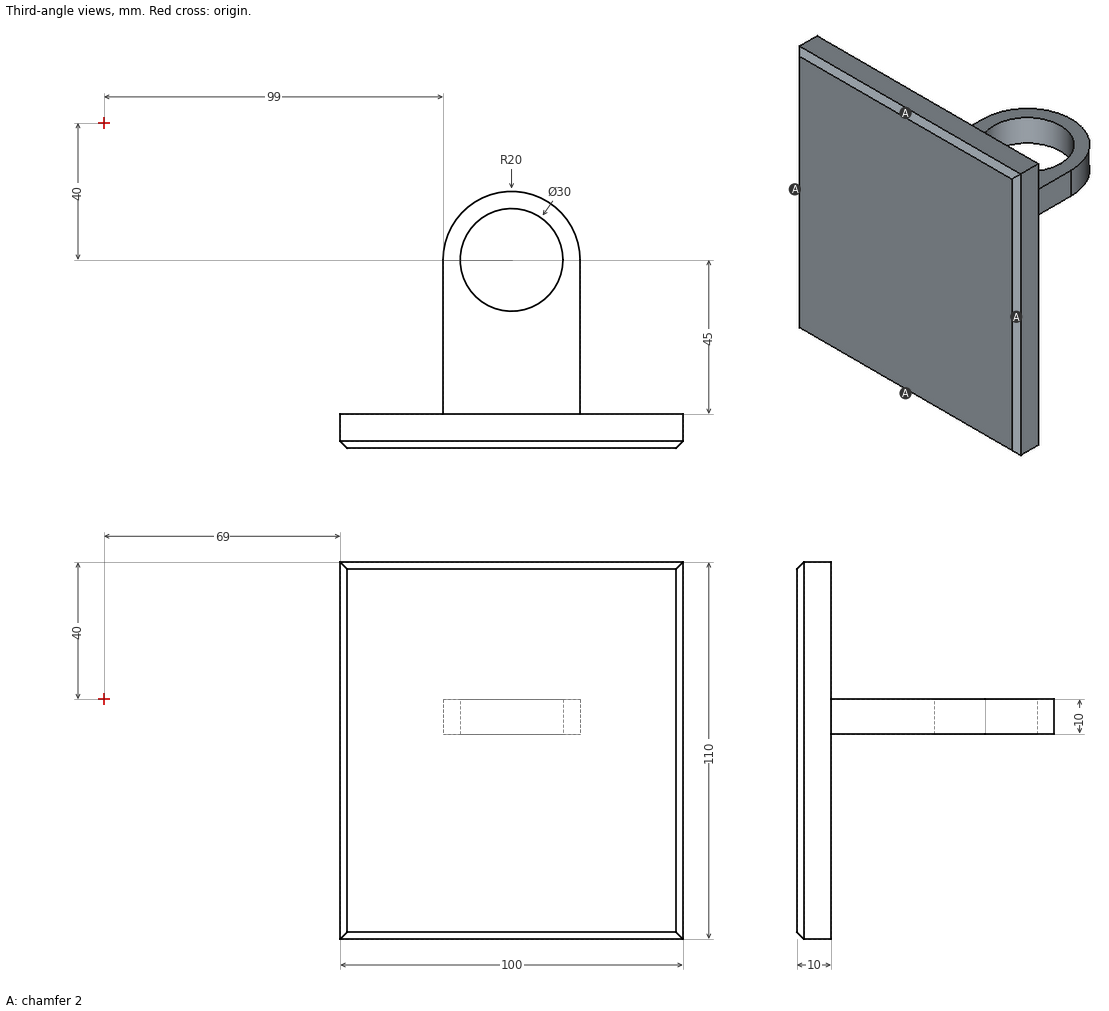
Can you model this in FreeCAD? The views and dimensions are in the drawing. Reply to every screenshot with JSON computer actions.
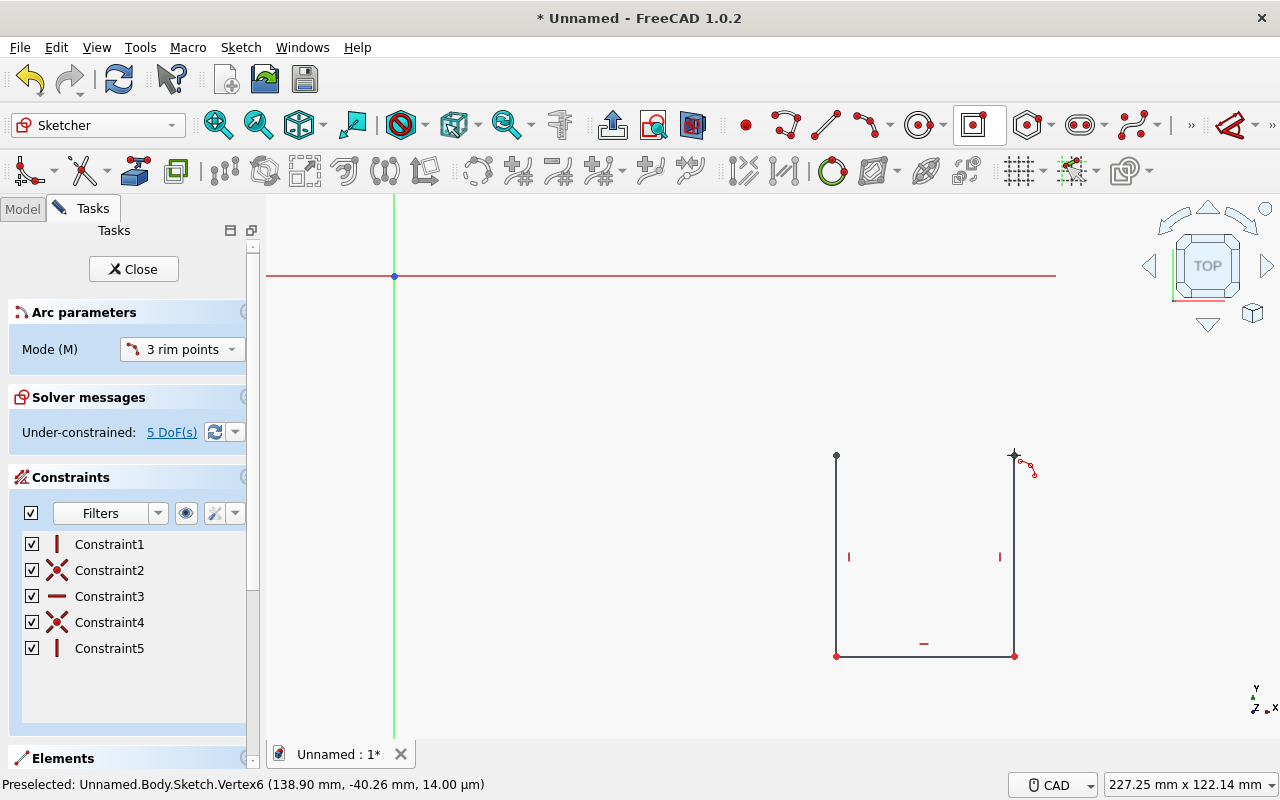
{"action": "left_click", "coordinate": [1014, 456]}
{"action": "left_click", "coordinate": [836, 456]}
{"action": "left_click", "coordinate": [925, 366]}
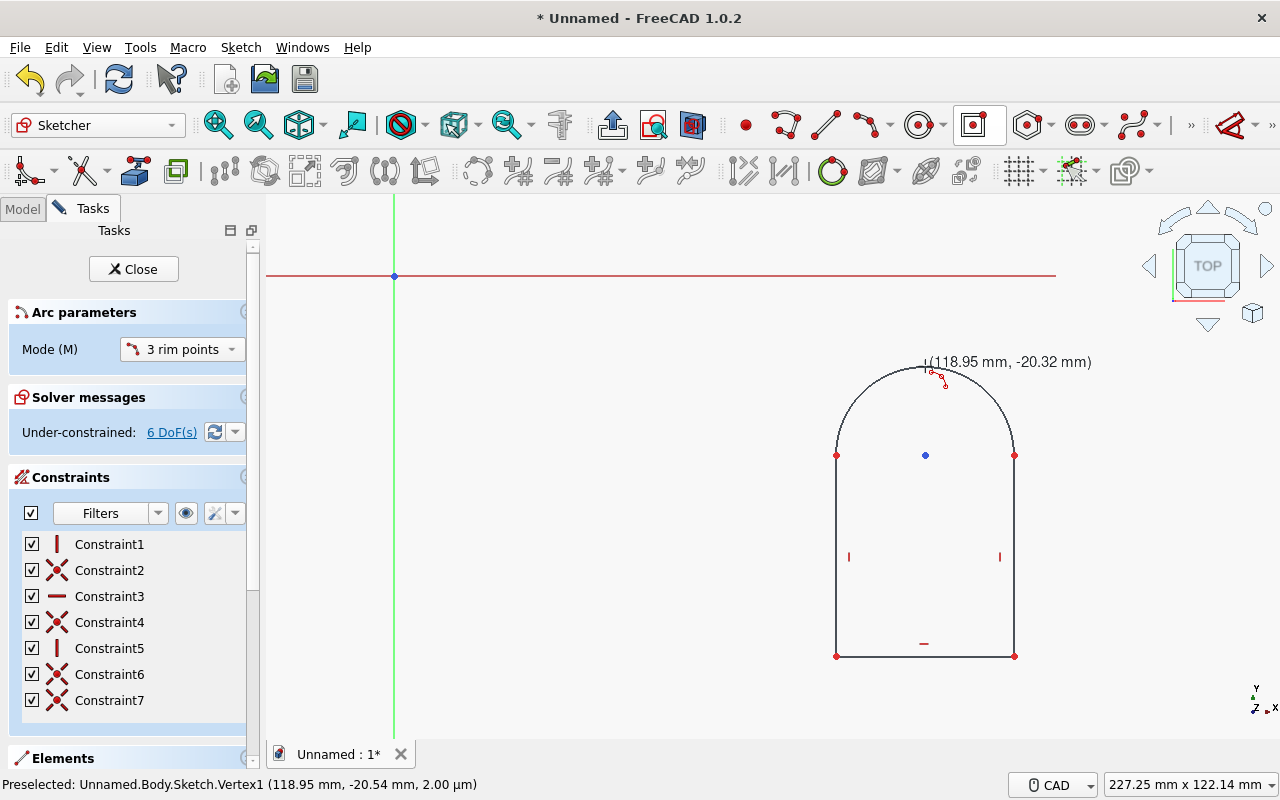
{"action": "left_click", "coordinate": [920, 126]}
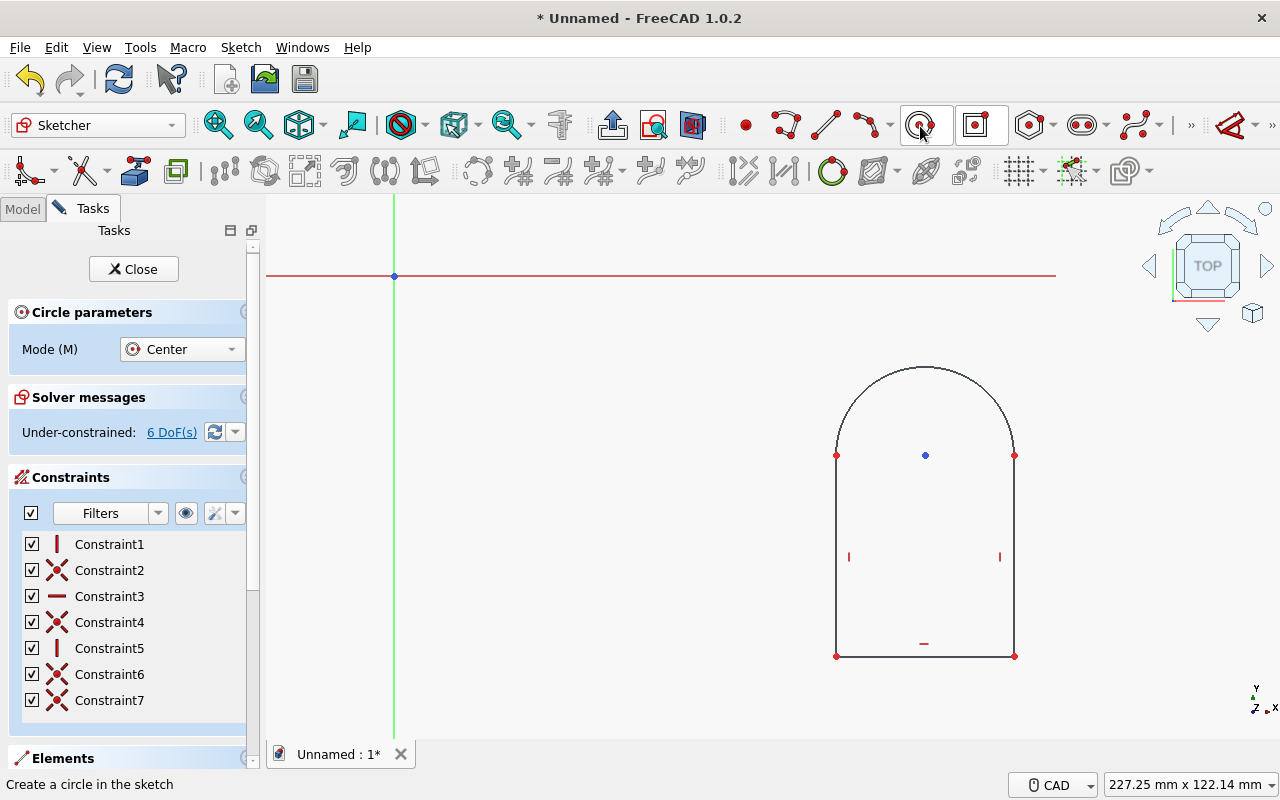
{"action": "left_click", "coordinate": [925, 455]}
{"action": "mouse_move", "coordinate": [973, 407]}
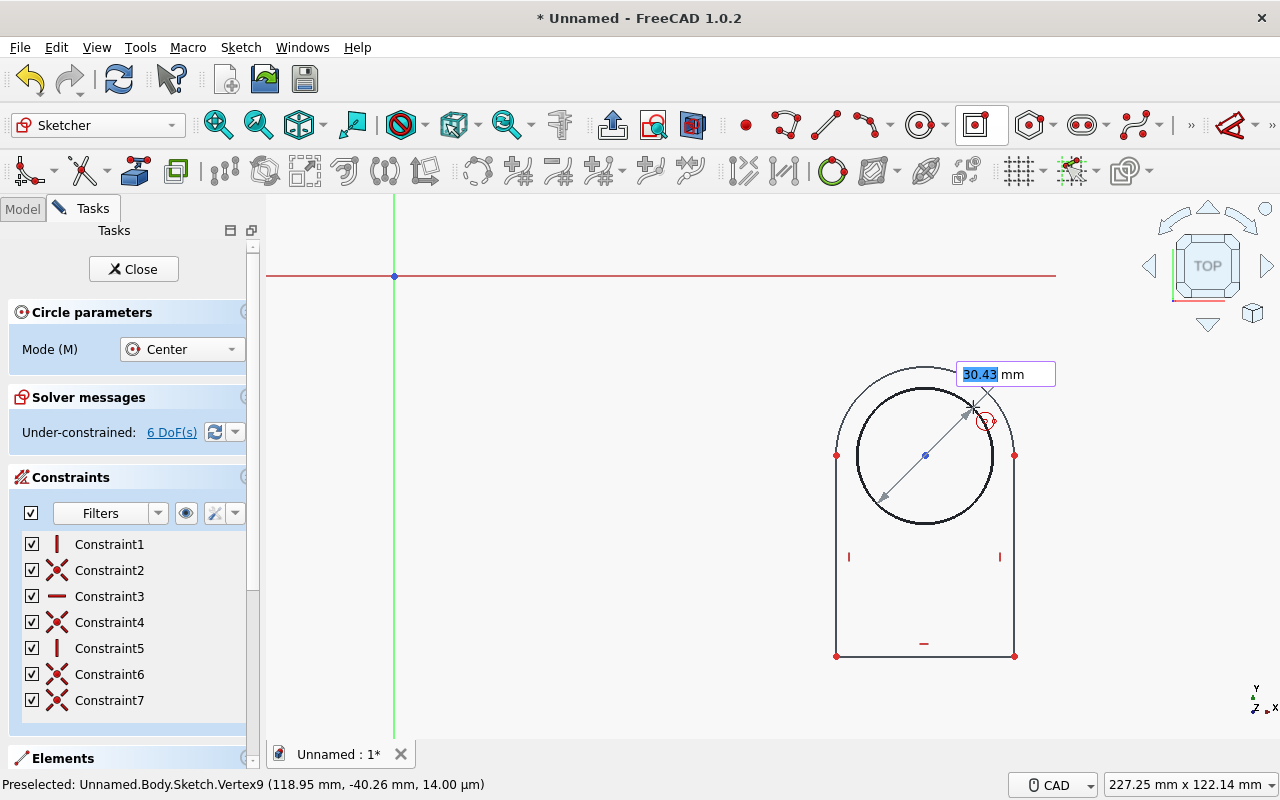
{"action": "type", "text": "30"}
{"action": "key", "text": "Return"}
{"action": "key", "text": "Escape"}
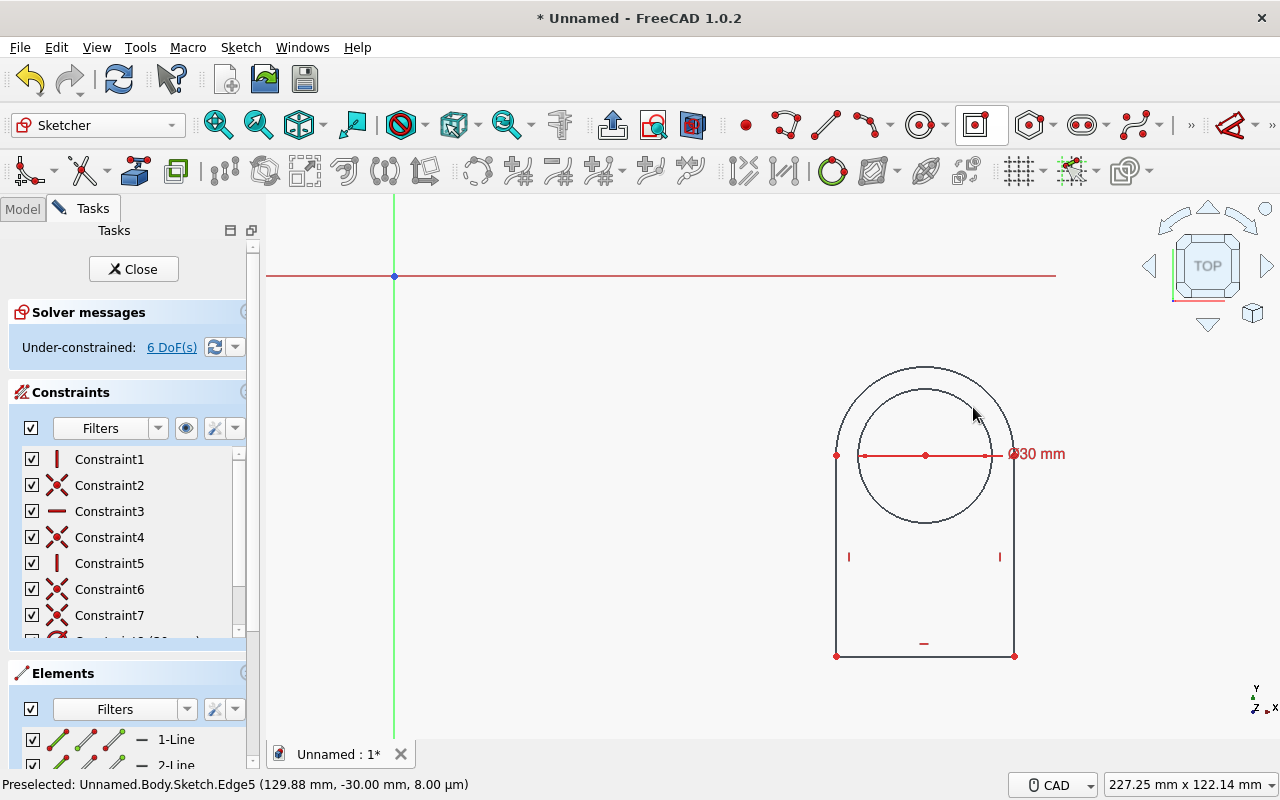
{"action": "left_click", "coordinate": [836, 516]}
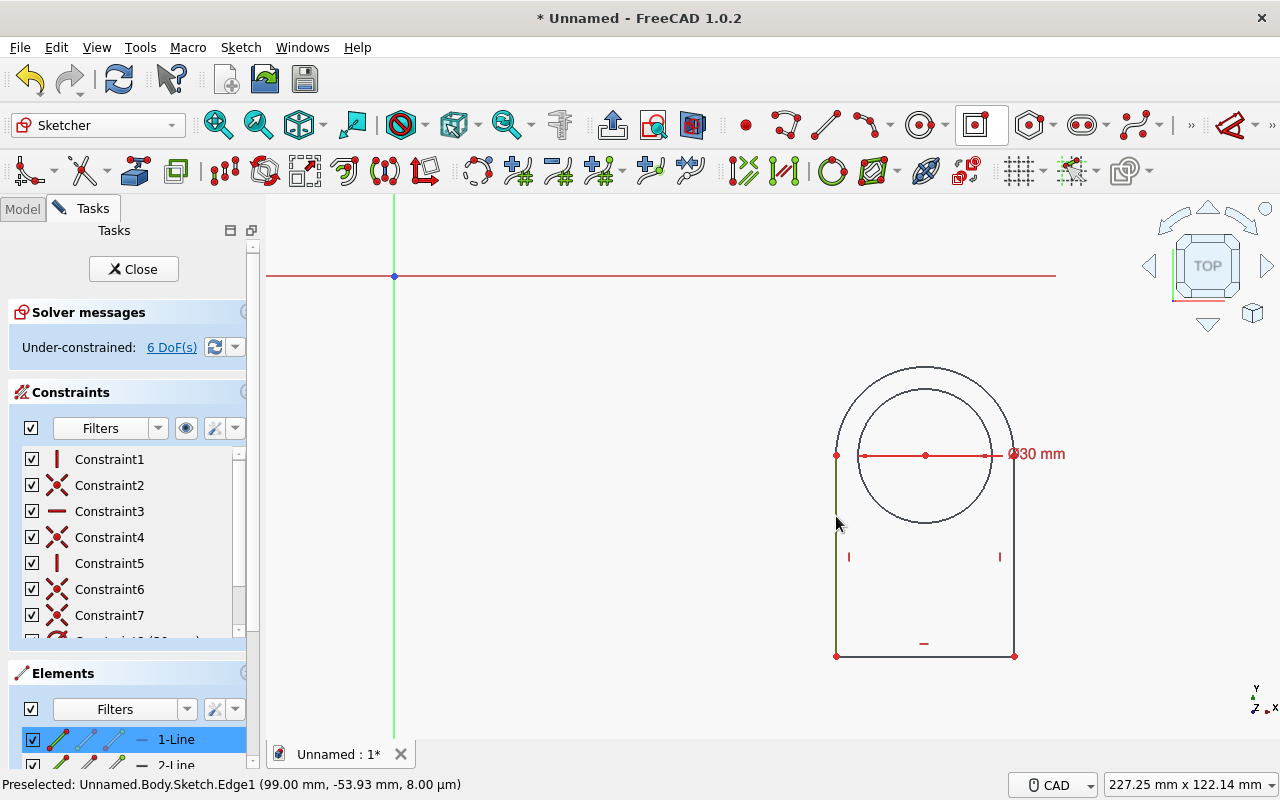
{"action": "left_click", "coordinate": [977, 384]}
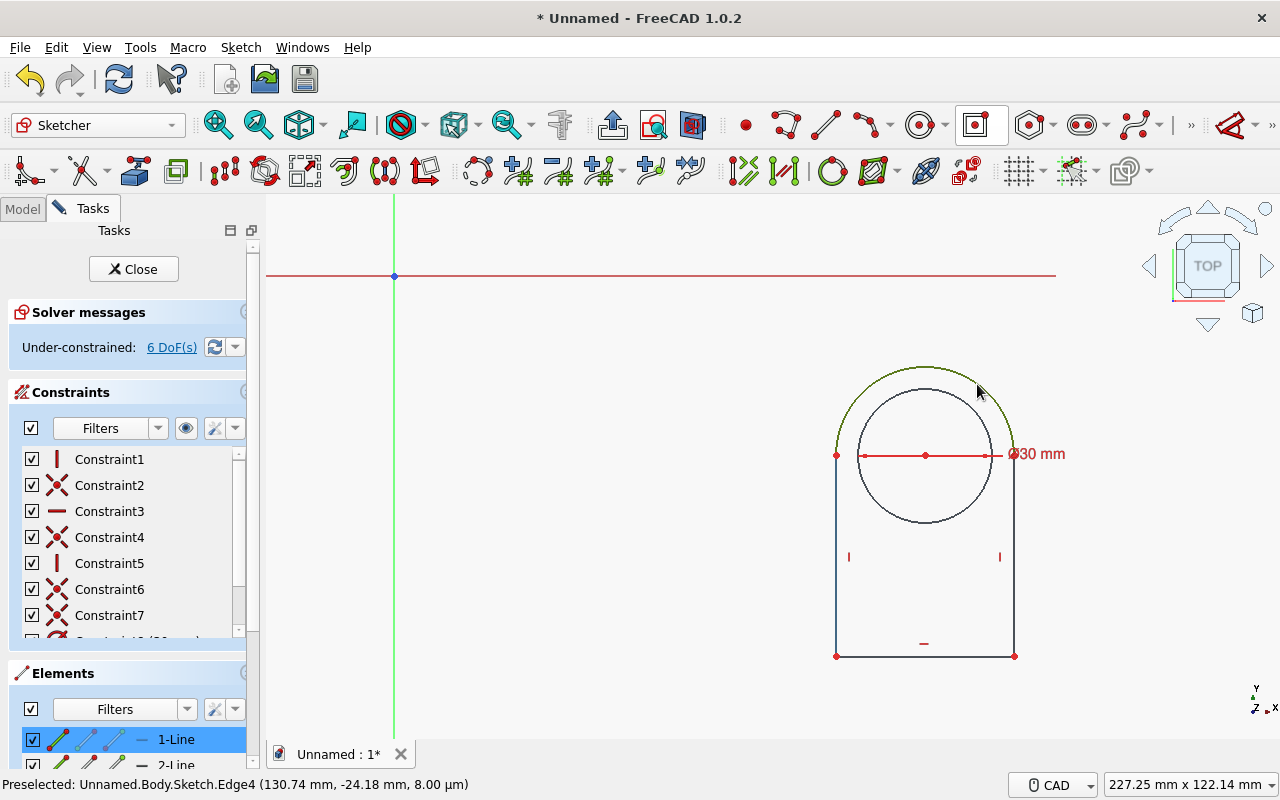
{"action": "key", "text": "t"}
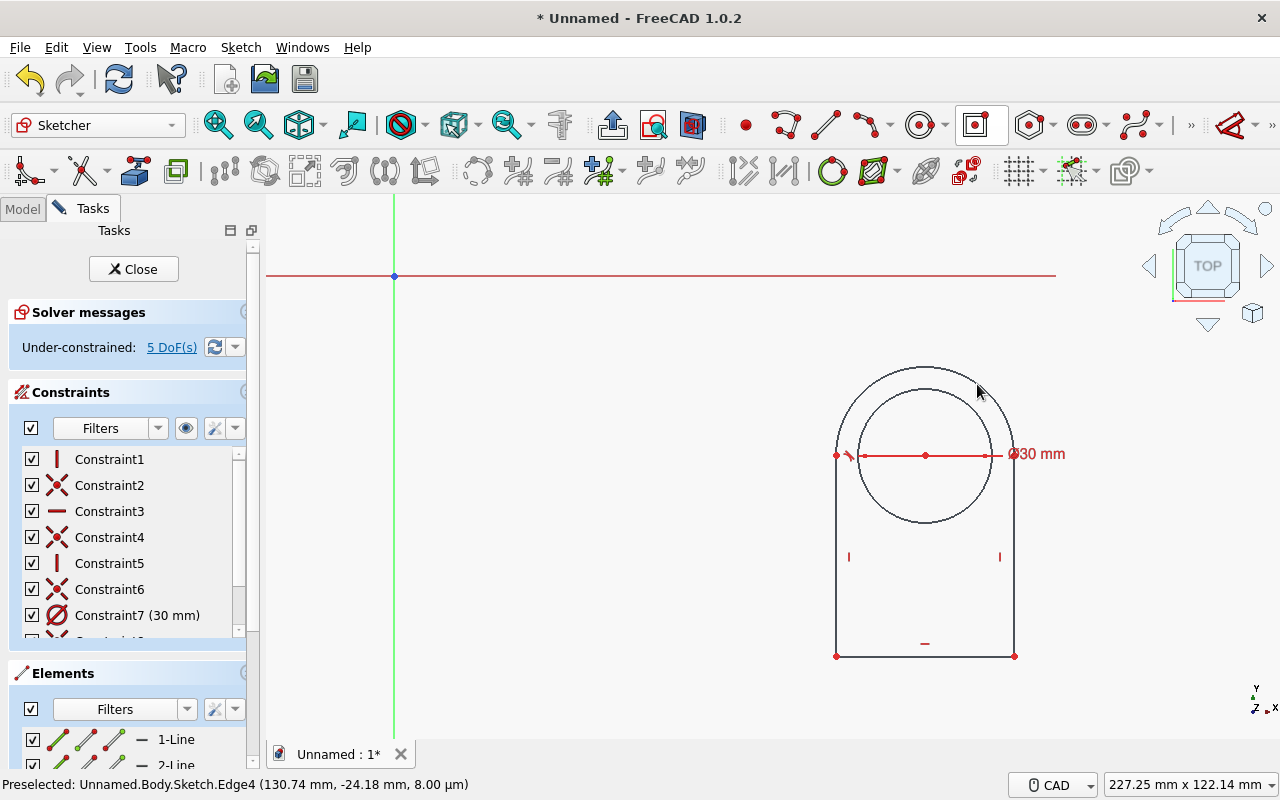
{"action": "left_click", "coordinate": [1014, 597]}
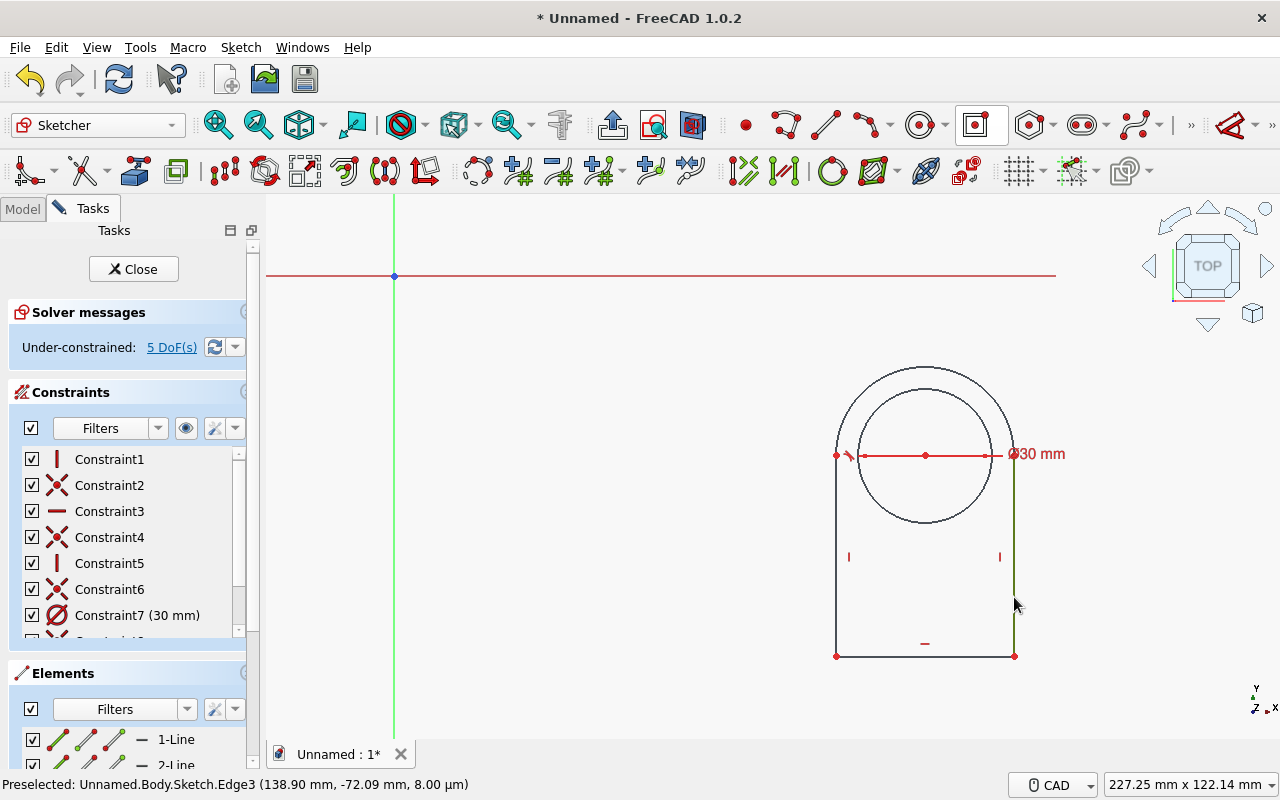
{"action": "left_click", "coordinate": [977, 384]}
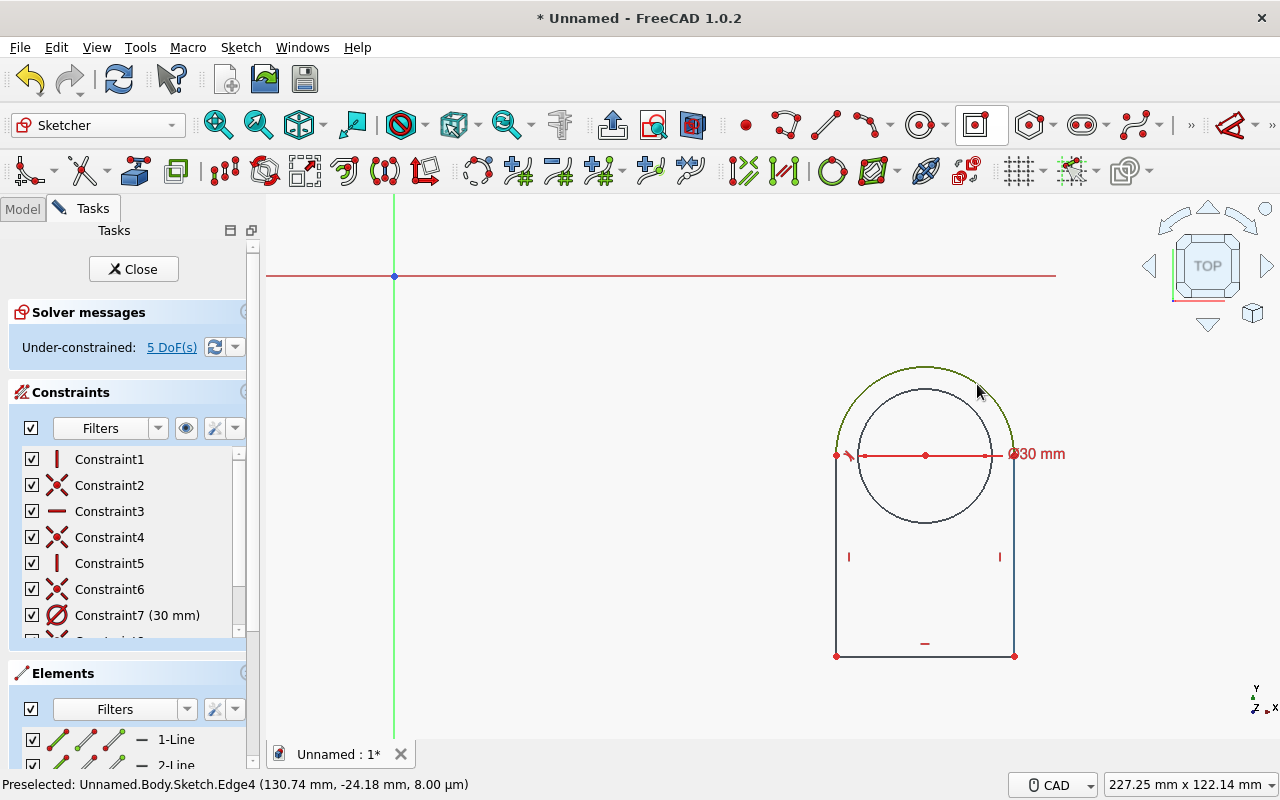
{"action": "key", "text": "t"}